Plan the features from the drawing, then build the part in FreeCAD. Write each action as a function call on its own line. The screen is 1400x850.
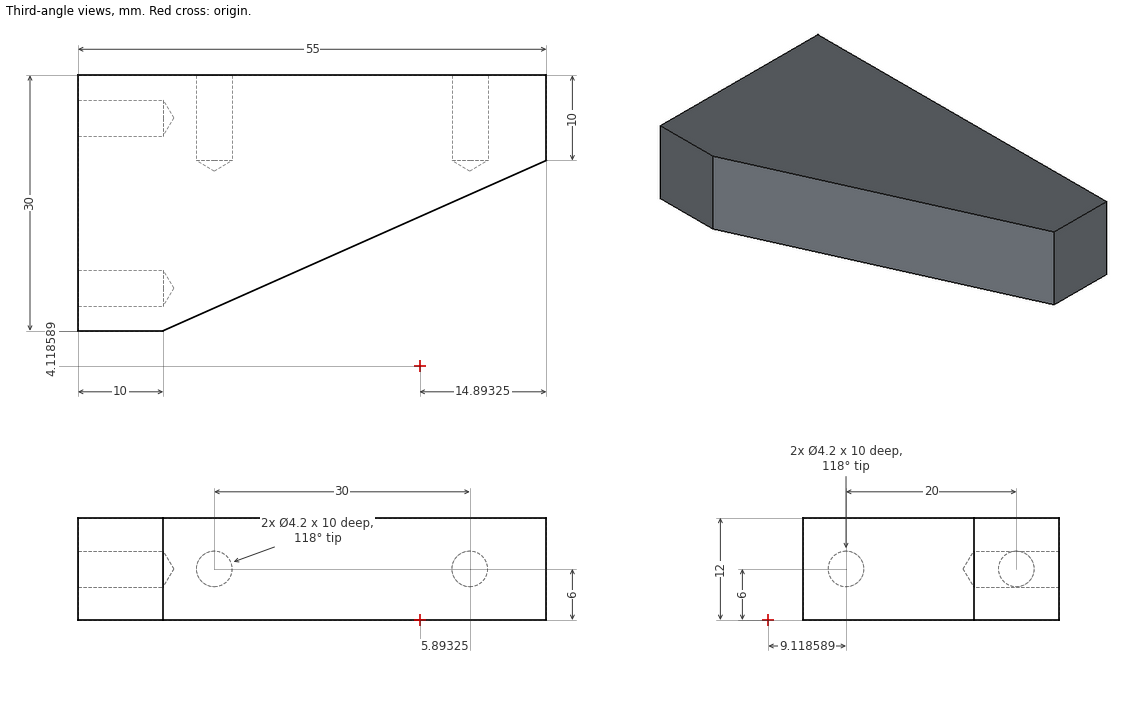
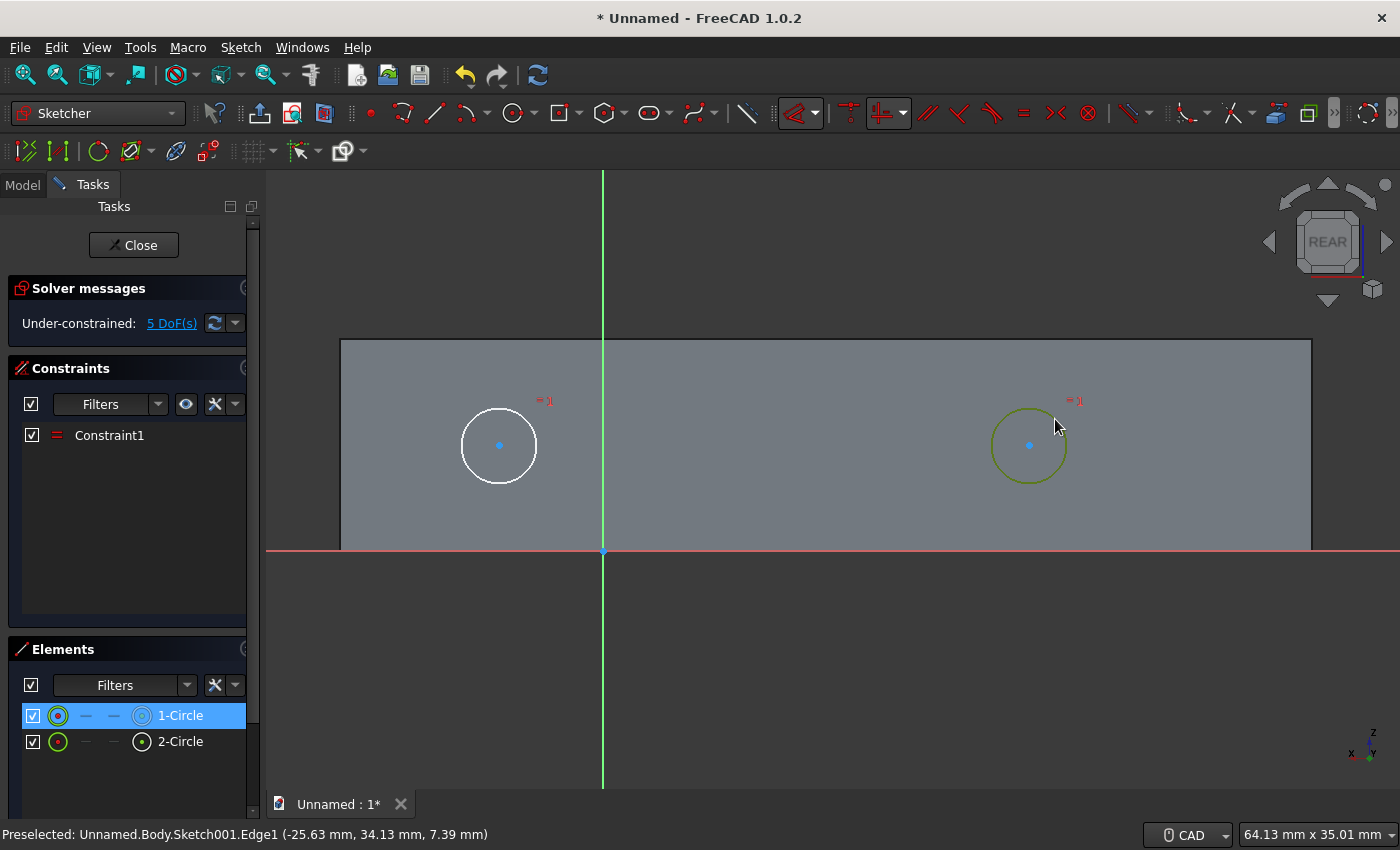
click(818, 114)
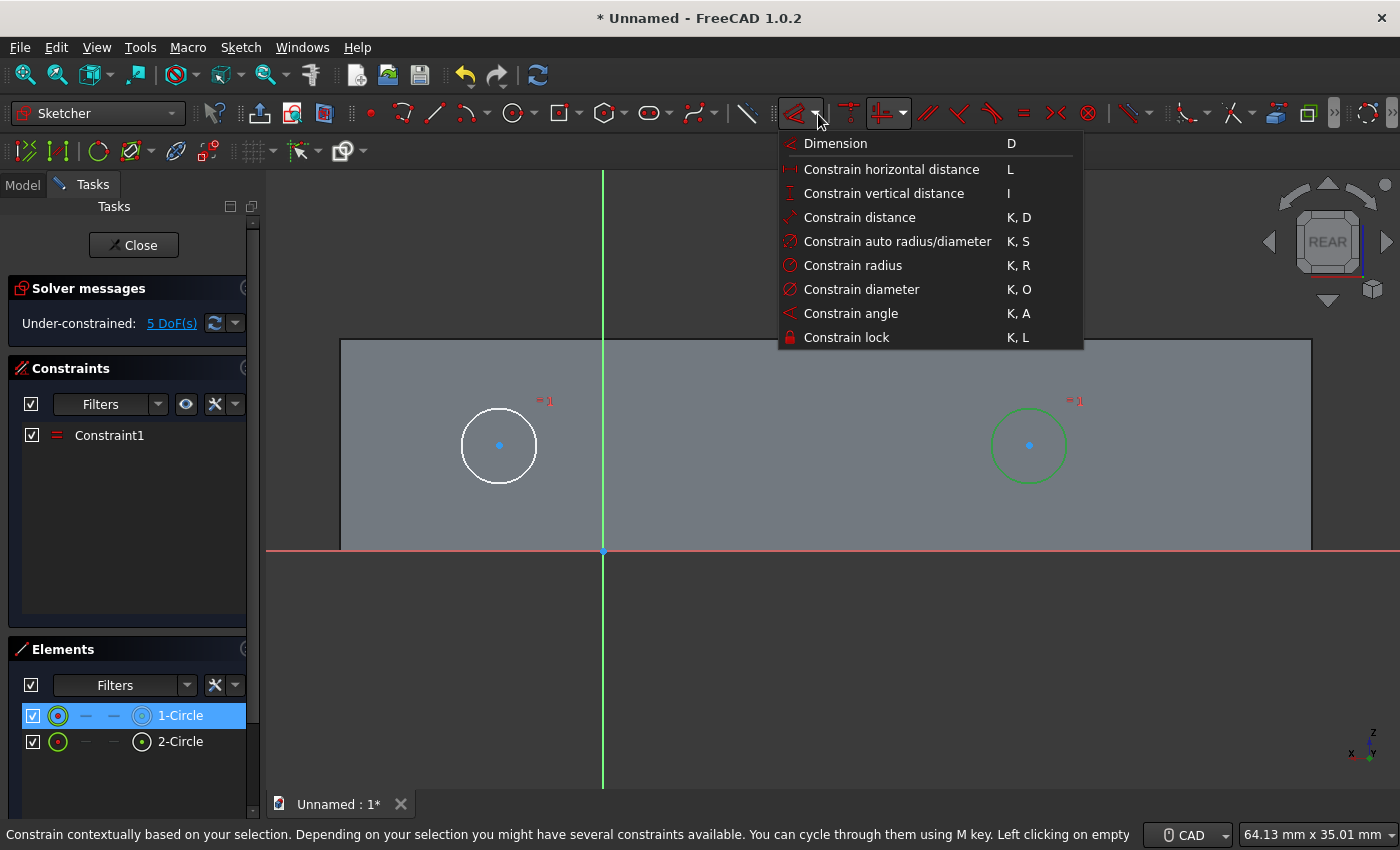
click(931, 289)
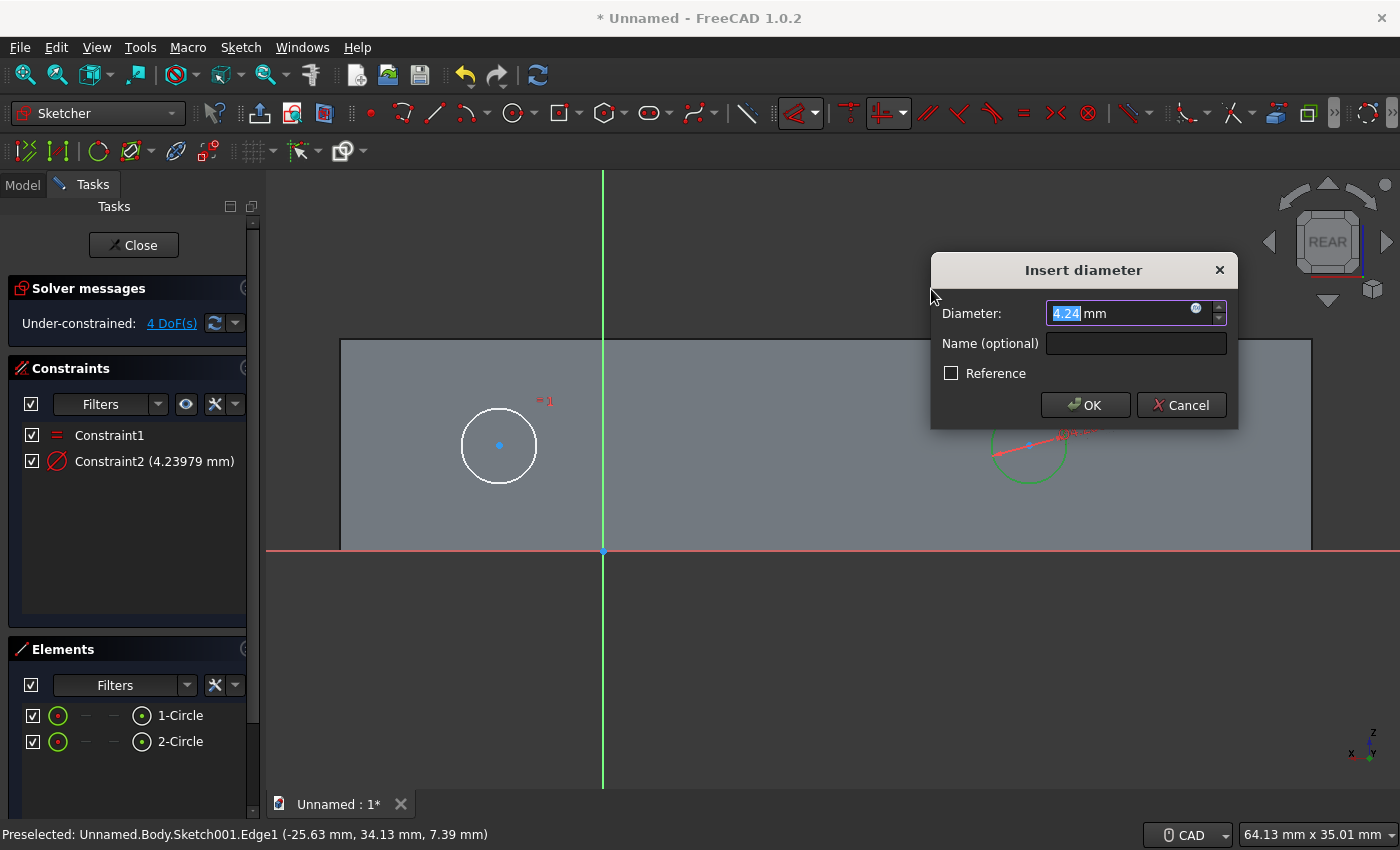
text(4.2)
key(Return)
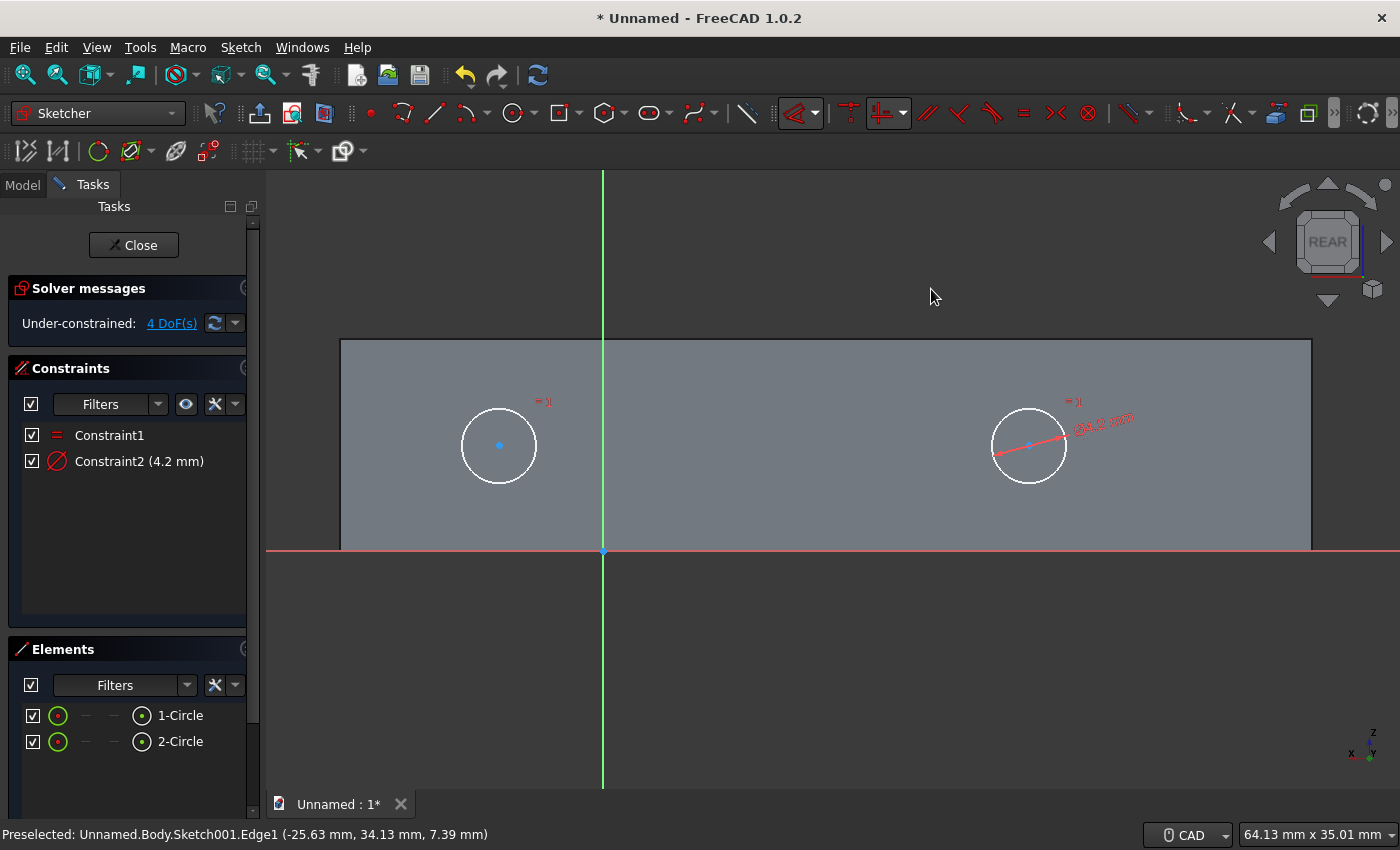
click(1029, 446)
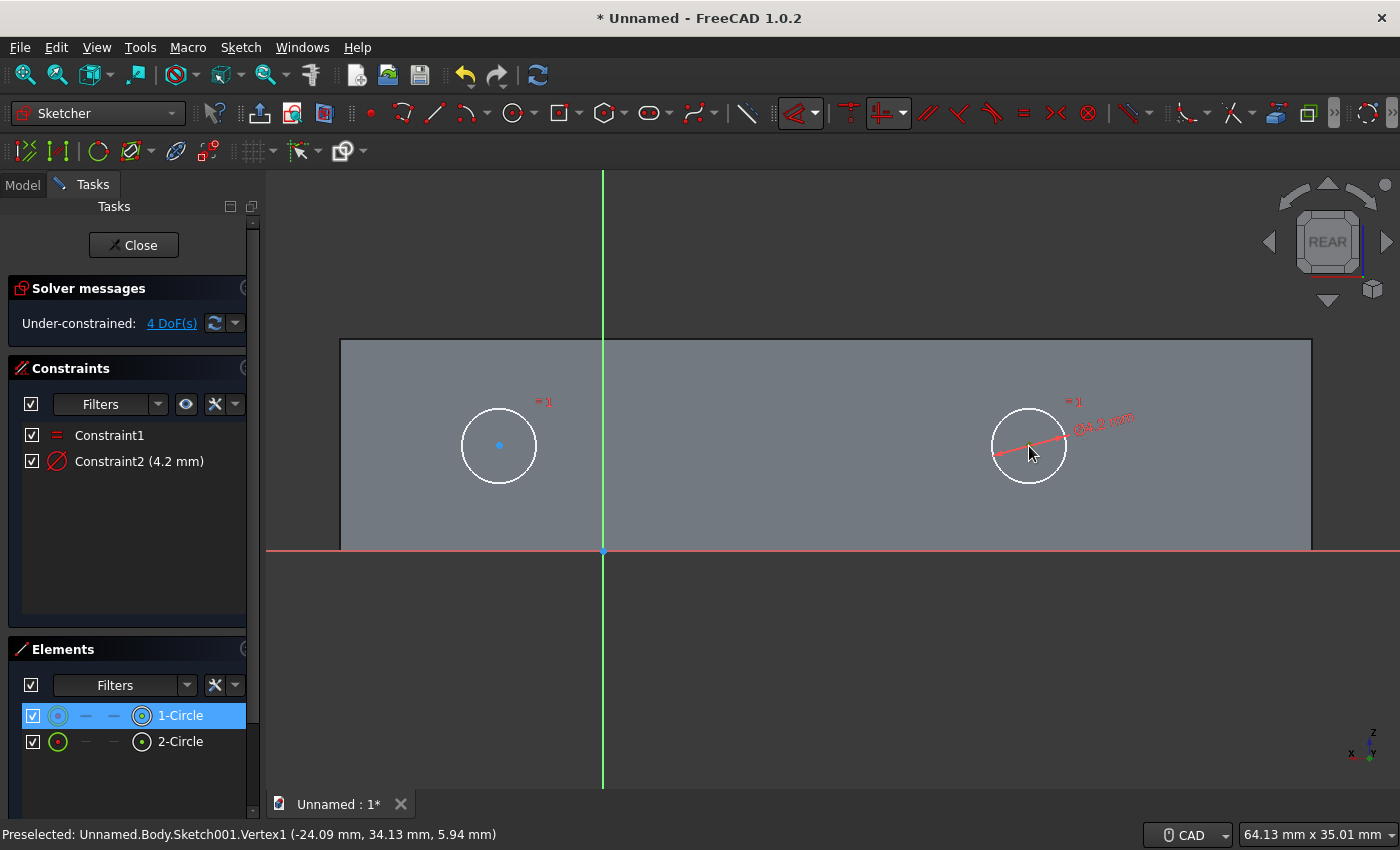
click(818, 114)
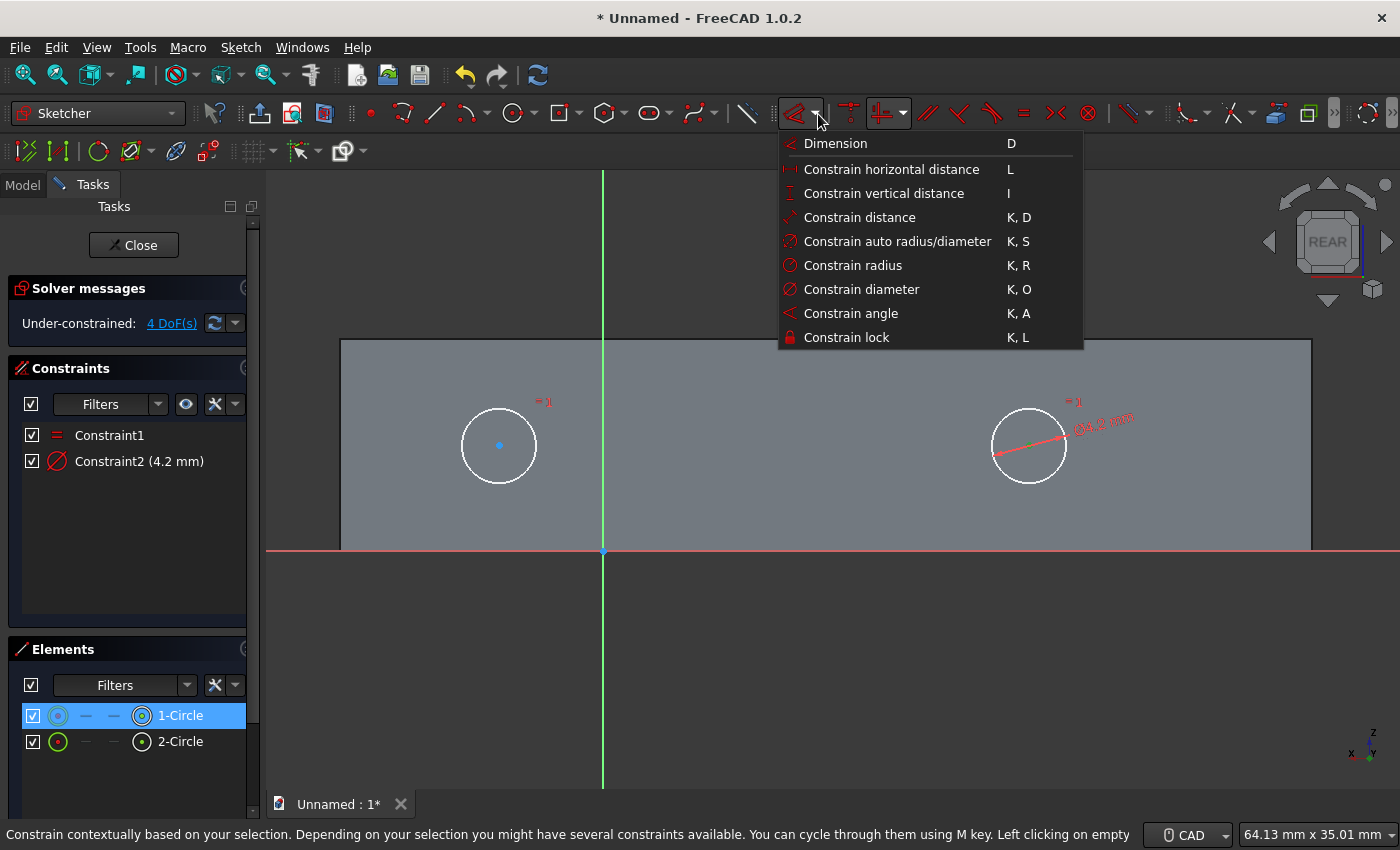
click(931, 193)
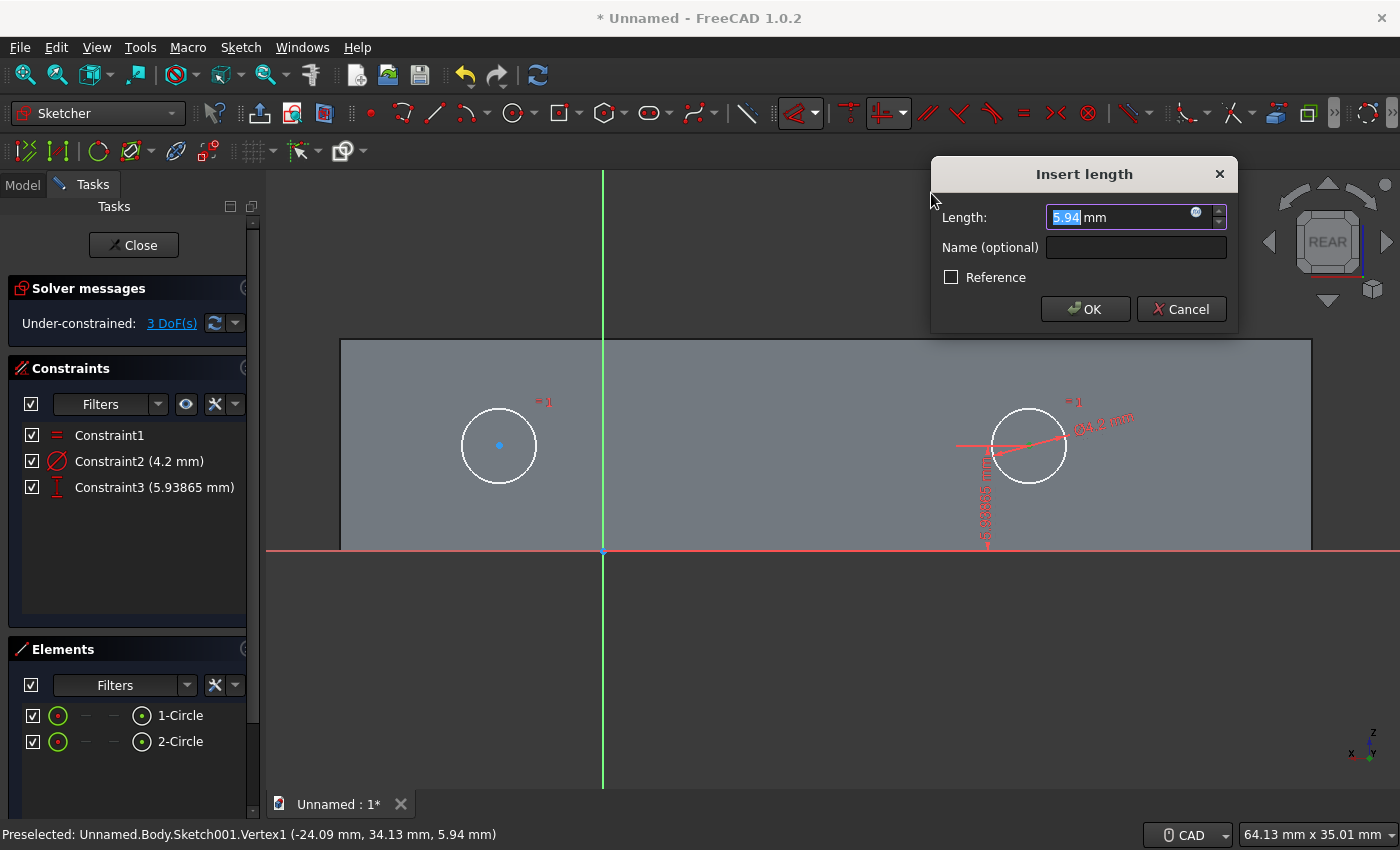
text(6)
key(Return)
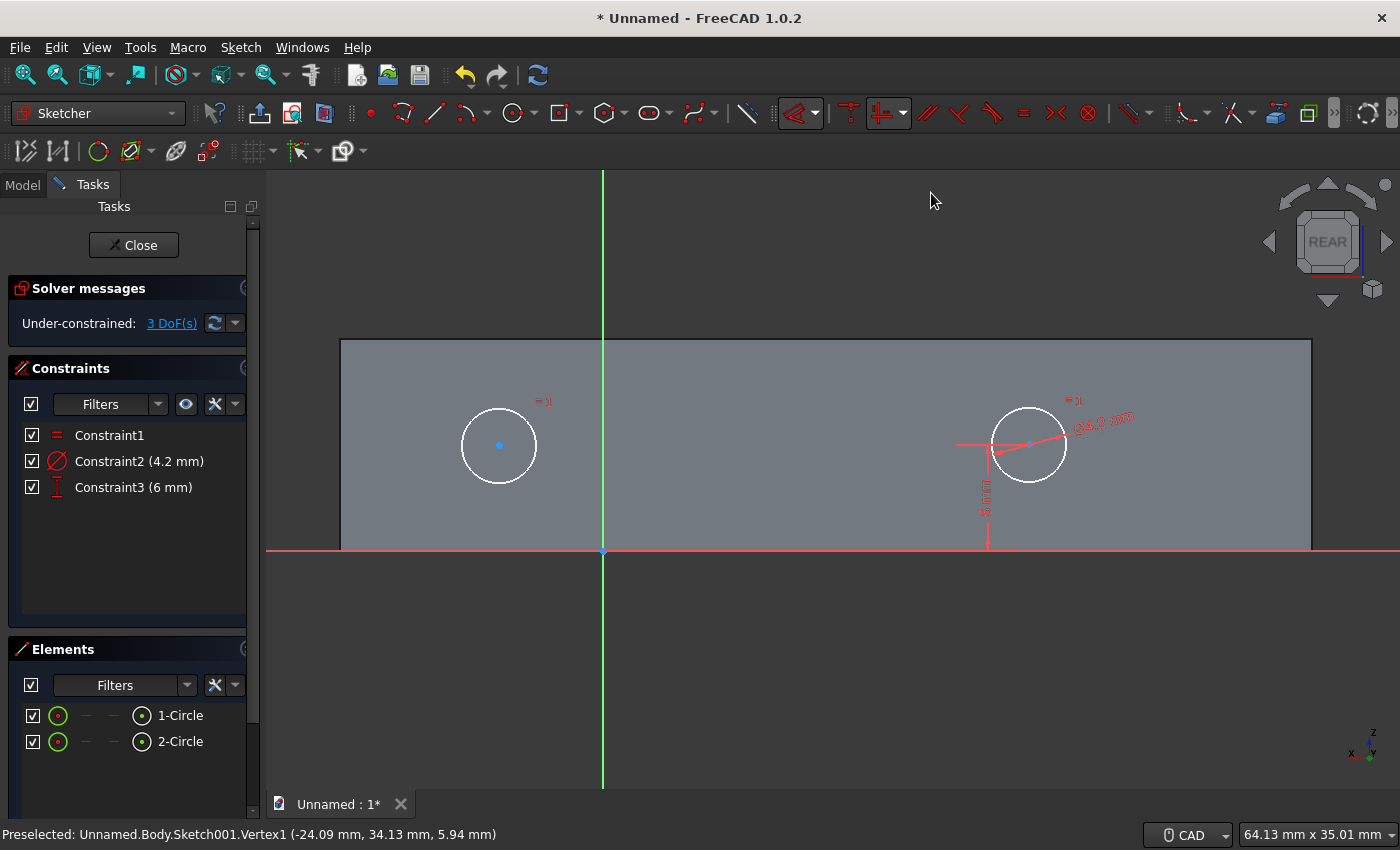
click(499, 446)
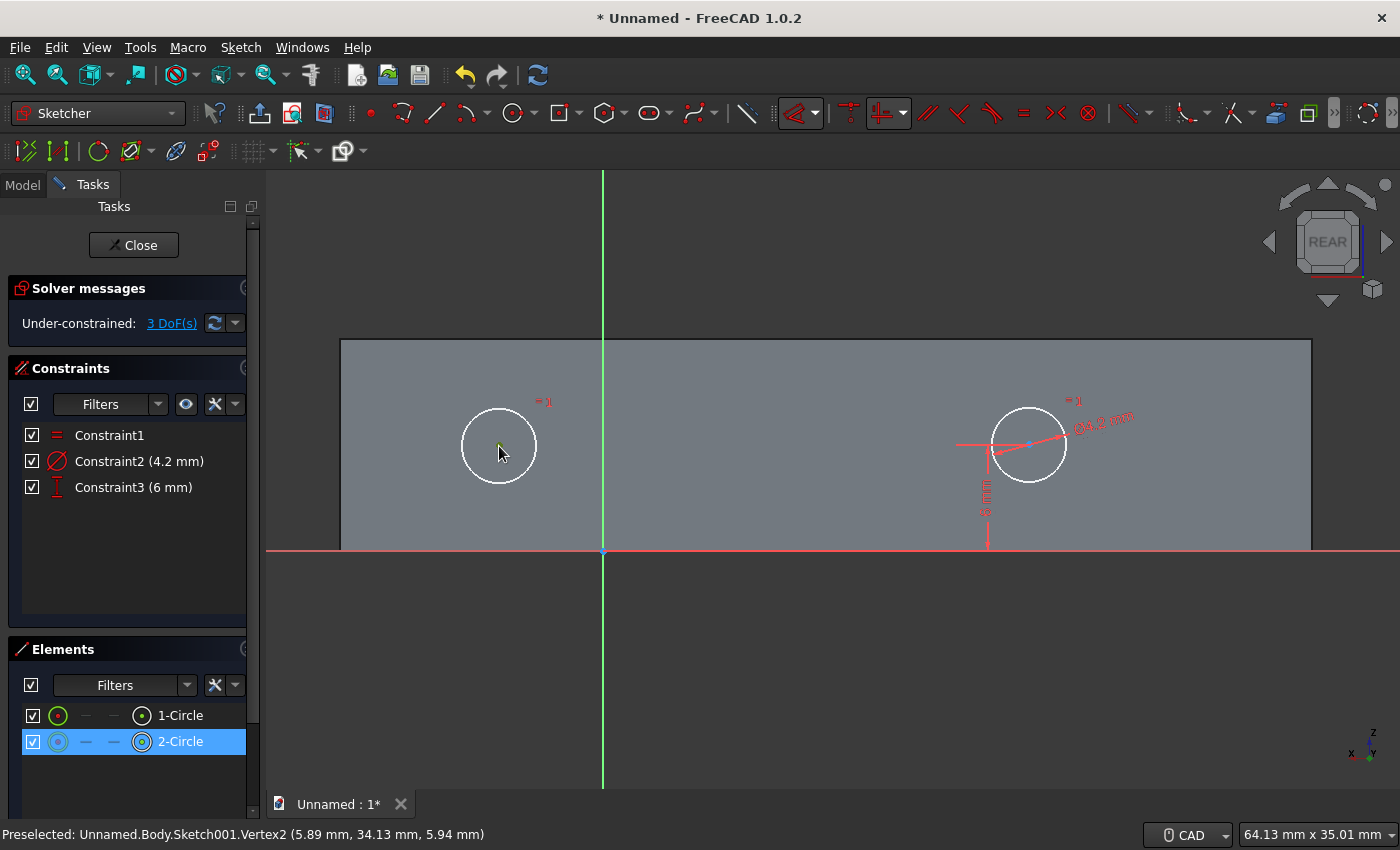
click(818, 114)